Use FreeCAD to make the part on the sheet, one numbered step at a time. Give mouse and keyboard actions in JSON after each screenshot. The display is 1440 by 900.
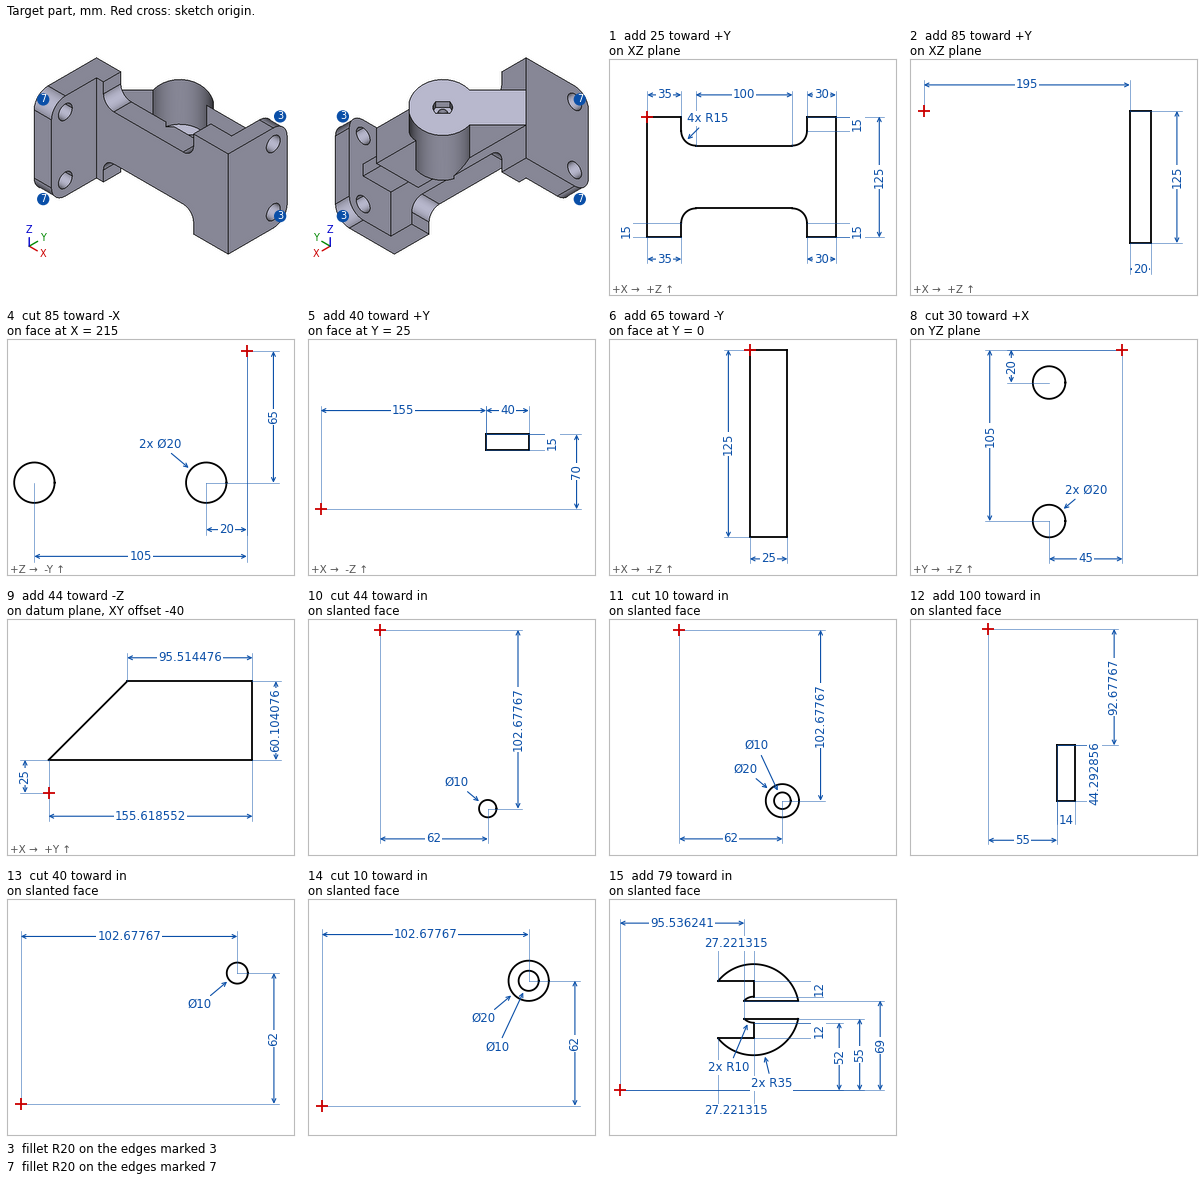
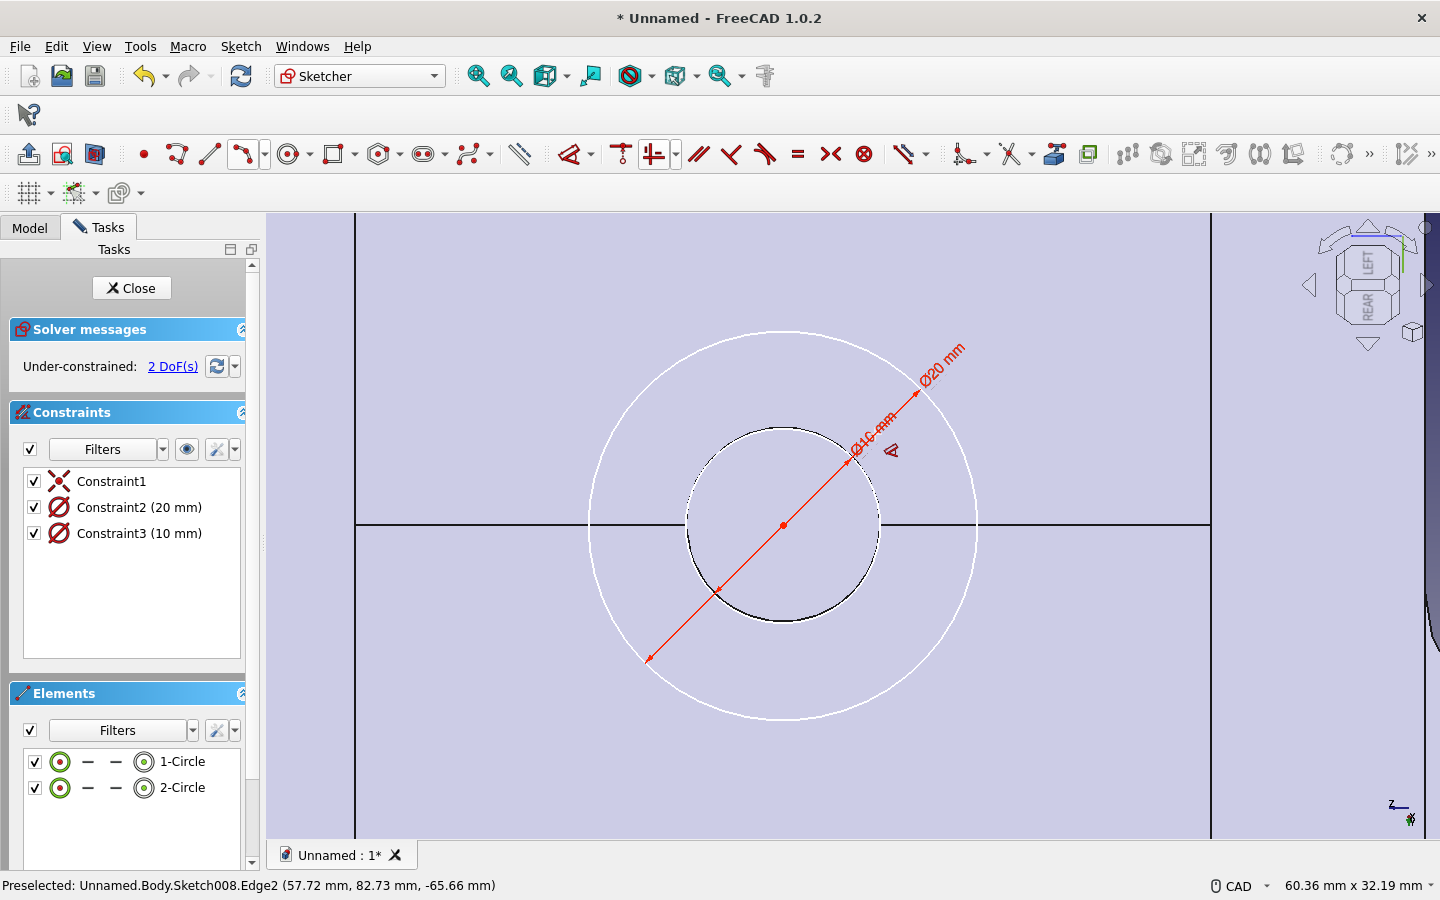
{"action": "left_click", "coordinate": [783, 526]}
{"action": "left_click", "coordinate": [539, 560]}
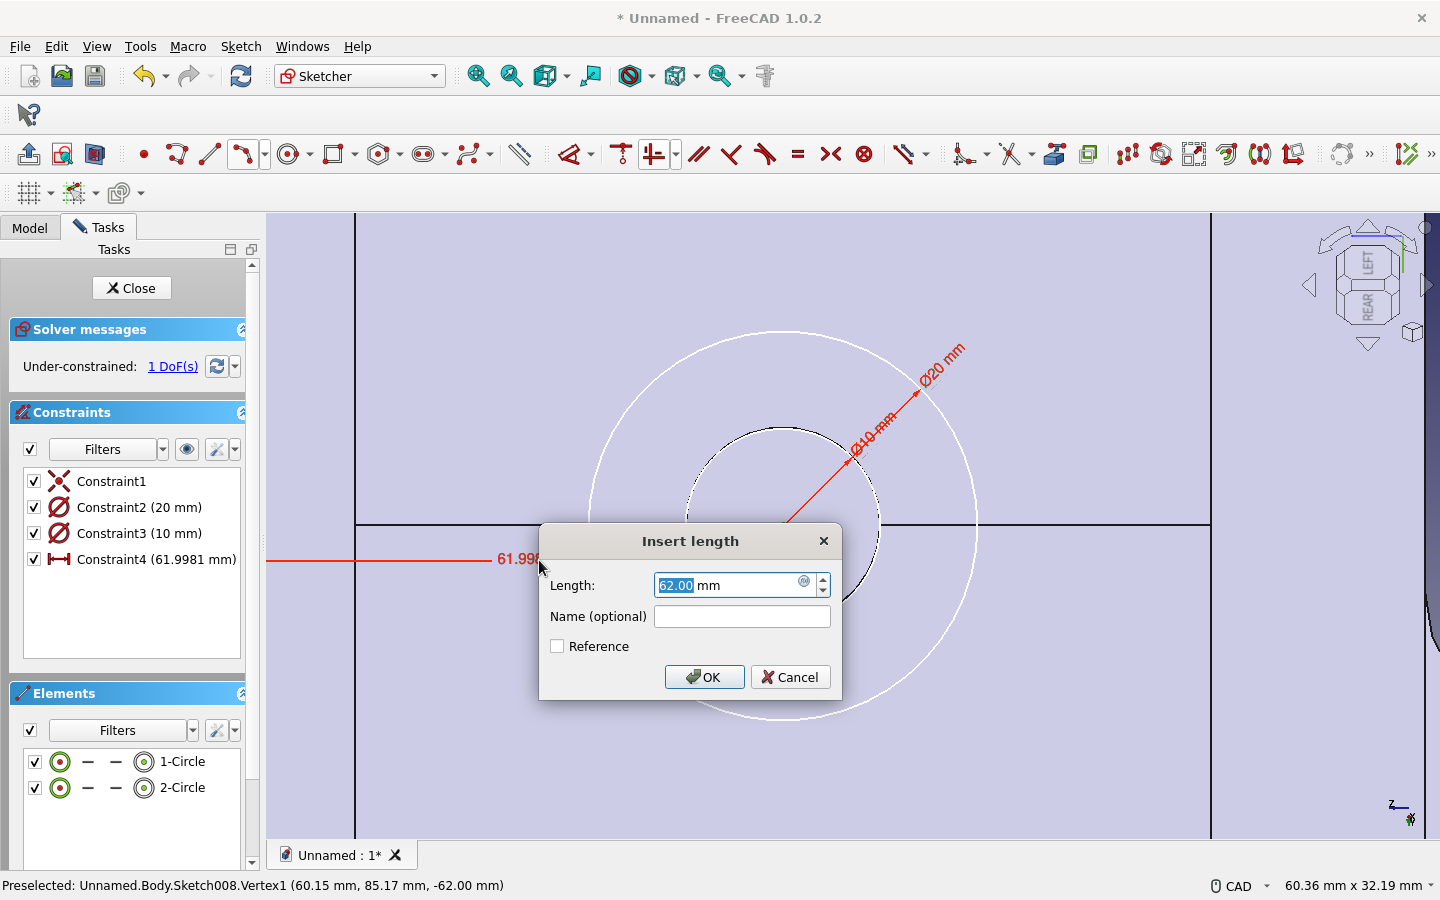
{"action": "type", "text": "62"}
{"action": "key", "text": "Return"}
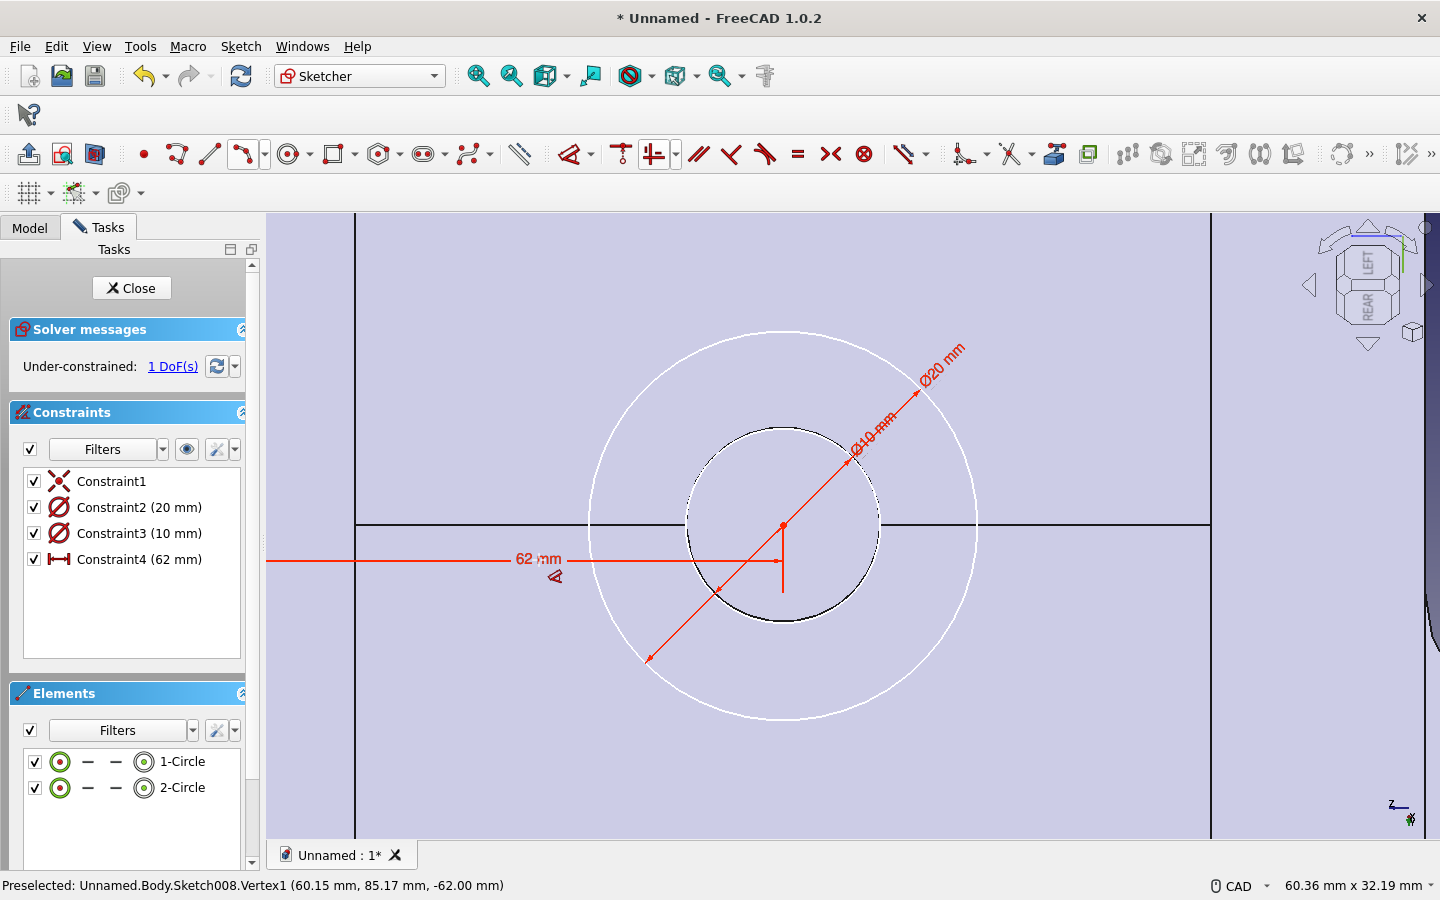
{"action": "left_click", "coordinate": [783, 526]}
{"action": "left_click", "coordinate": [817, 384]}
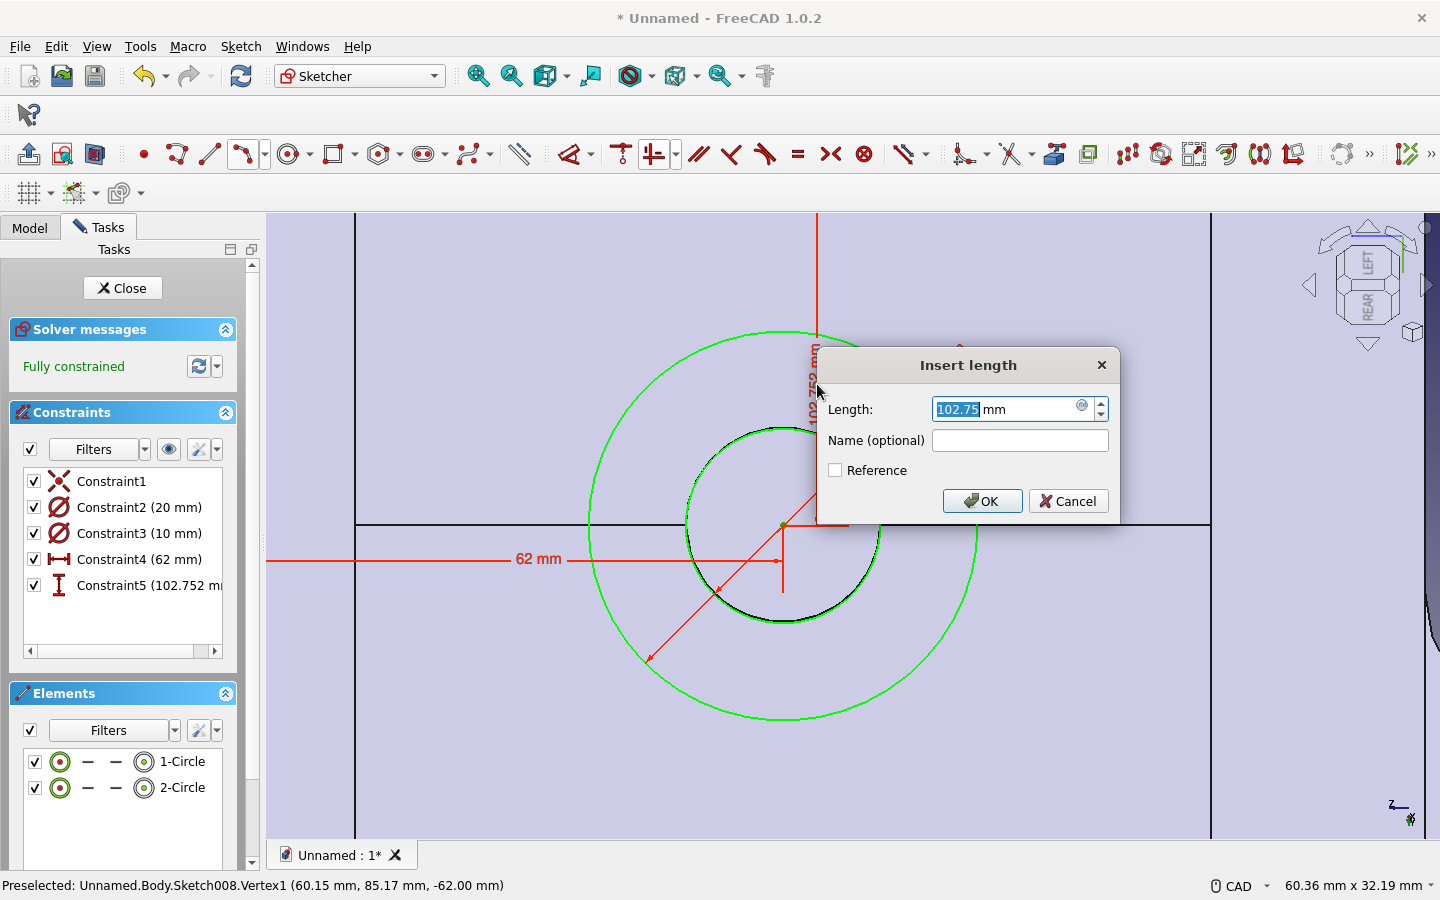
{"action": "type", "text": "102.67767"}
{"action": "key", "text": "Return"}
{"action": "key", "text": "Escape"}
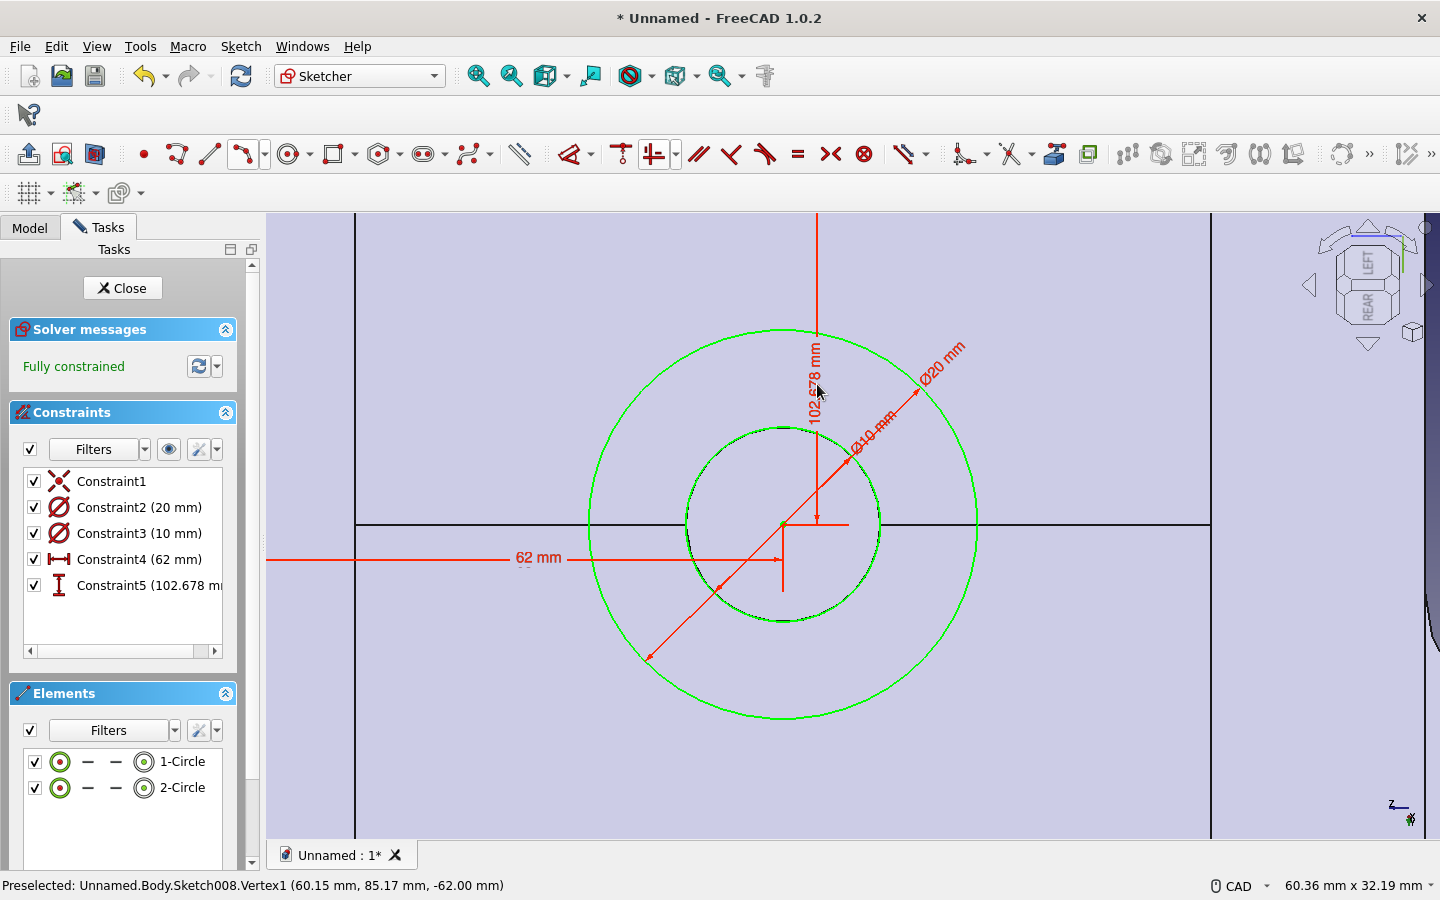
{"action": "left_click", "coordinate": [123, 288]}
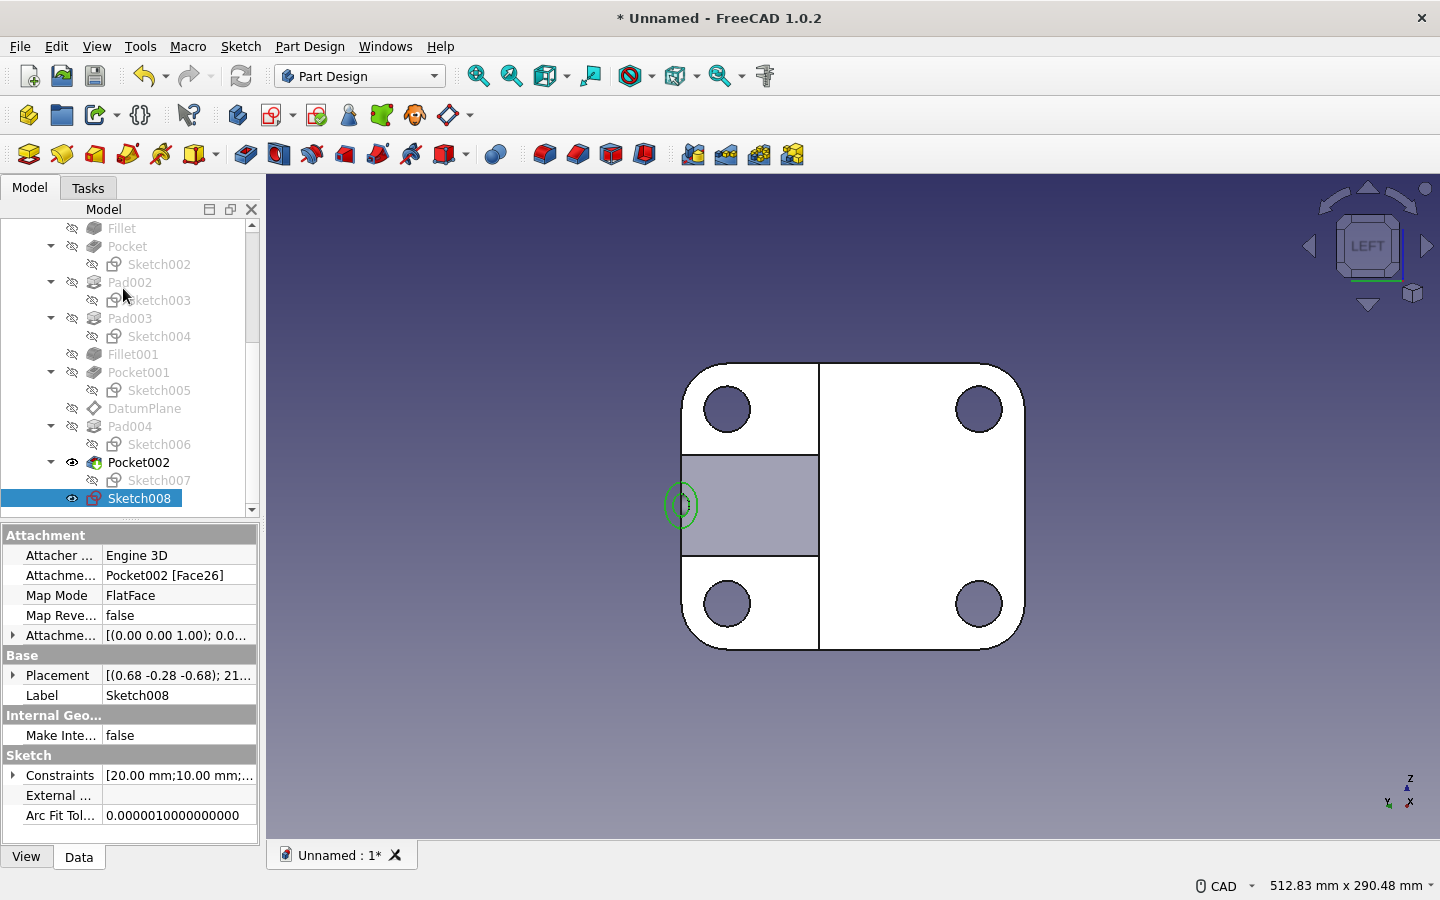
{"action": "left_click", "coordinate": [246, 154]}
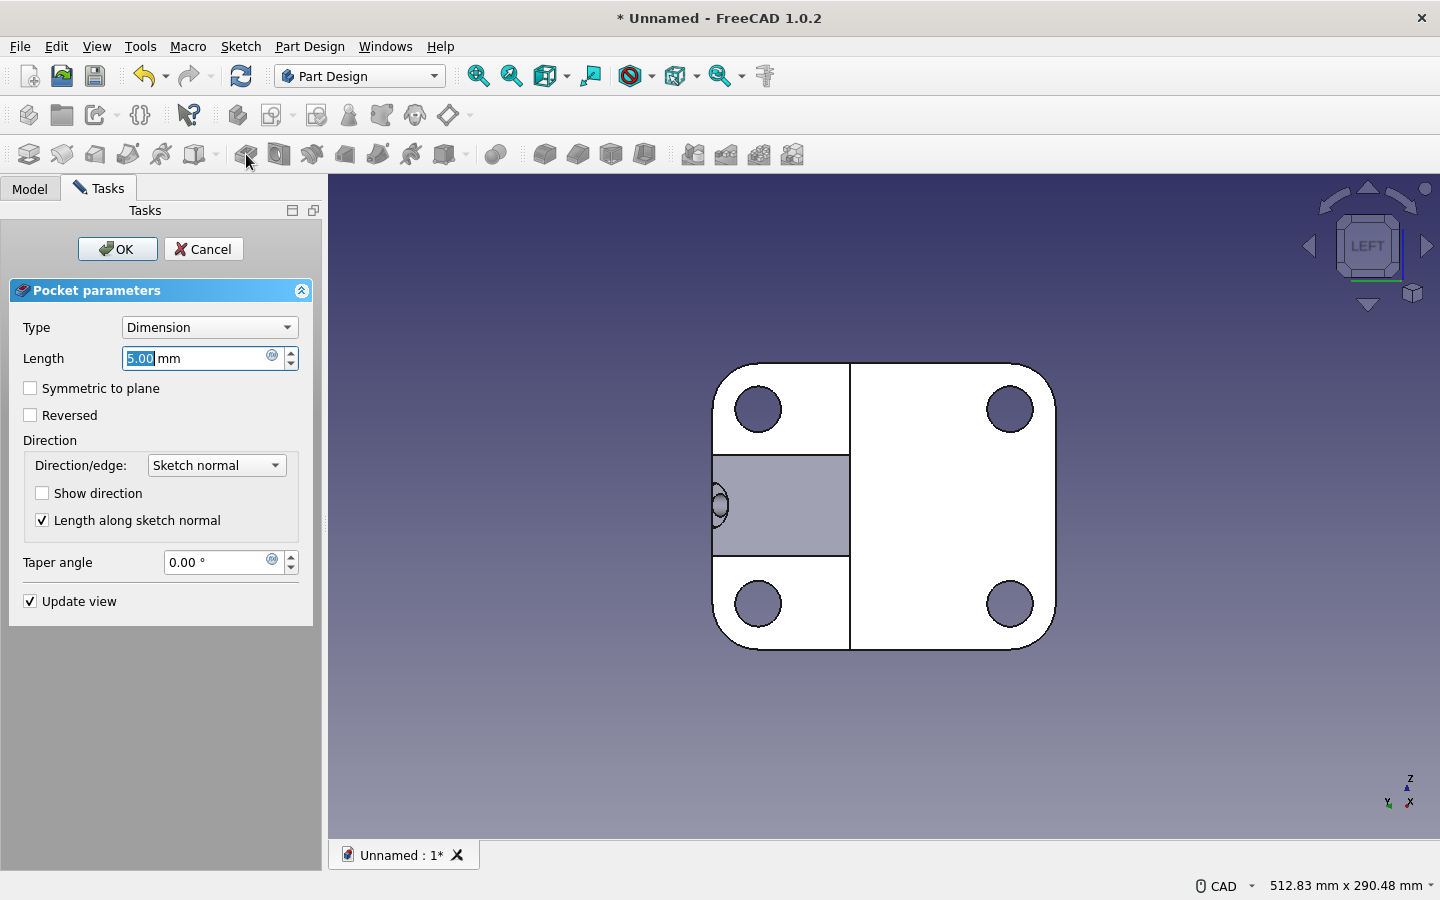
{"action": "type", "text": "10"}
{"action": "key", "text": "Tab"}